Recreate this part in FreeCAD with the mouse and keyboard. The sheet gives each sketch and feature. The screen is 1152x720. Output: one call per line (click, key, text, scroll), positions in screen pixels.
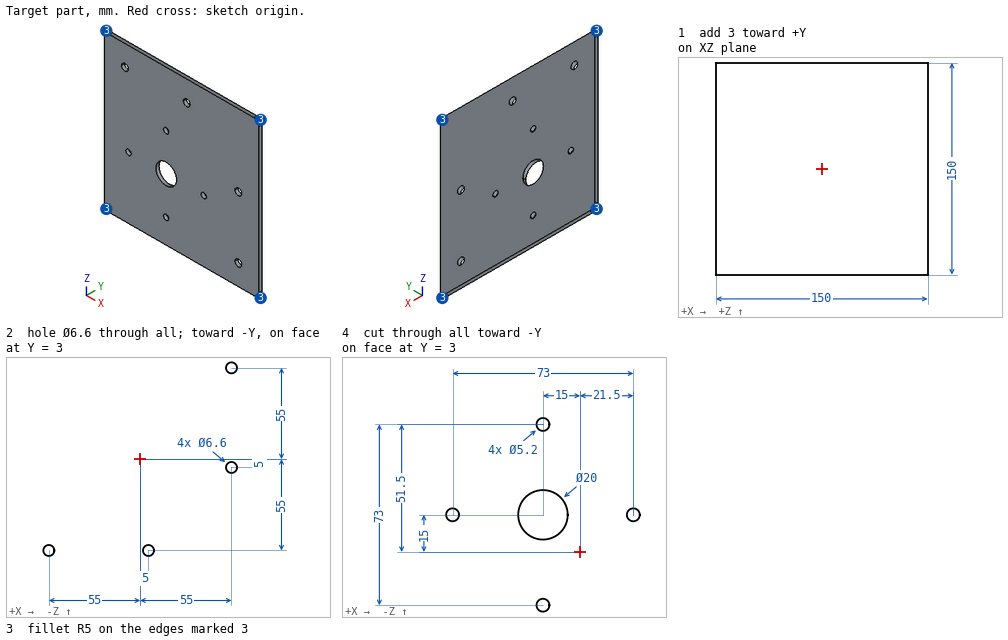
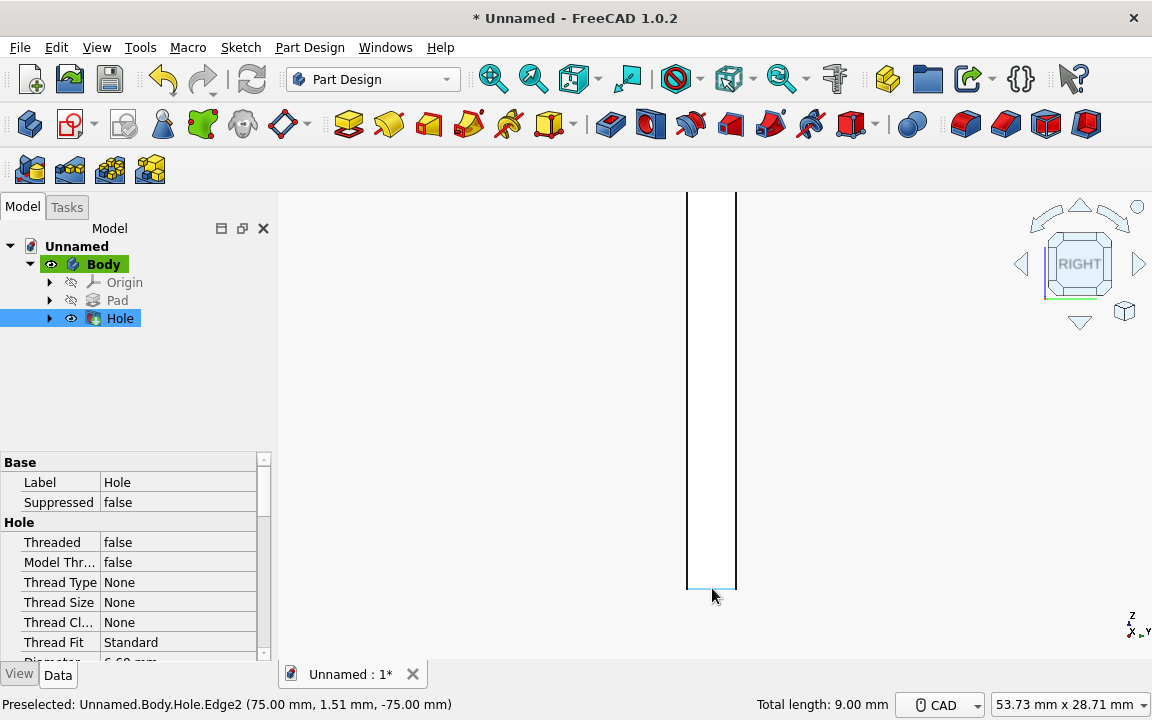
click(494, 80)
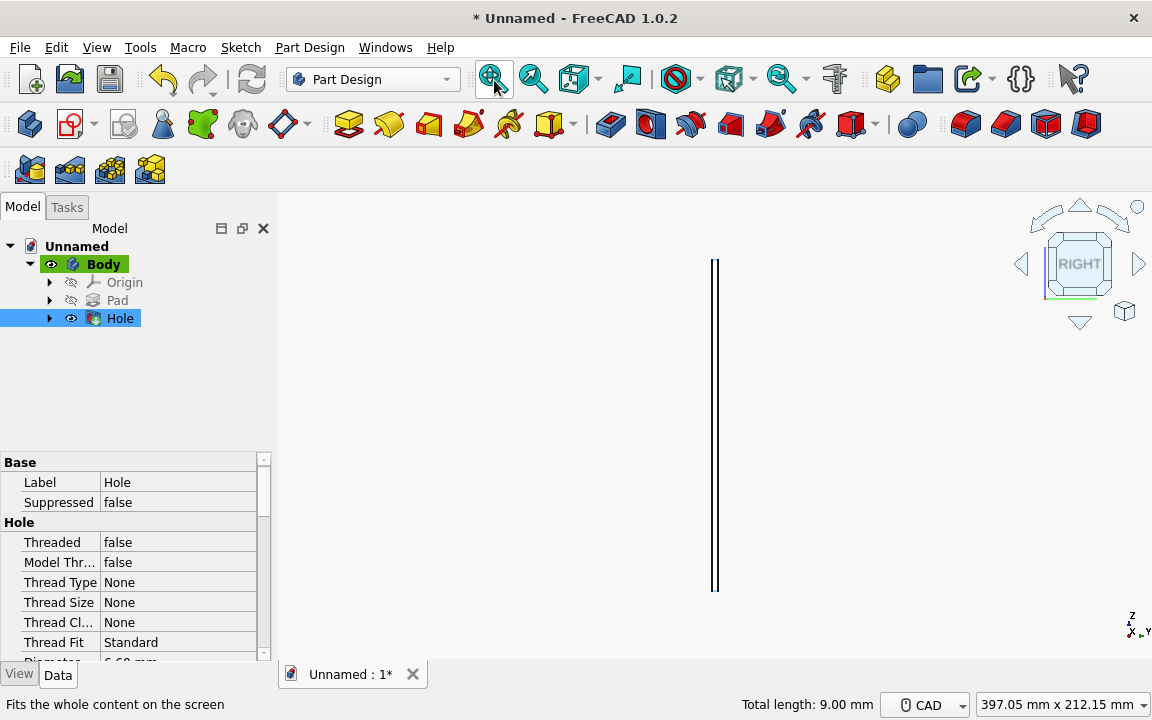
key(5)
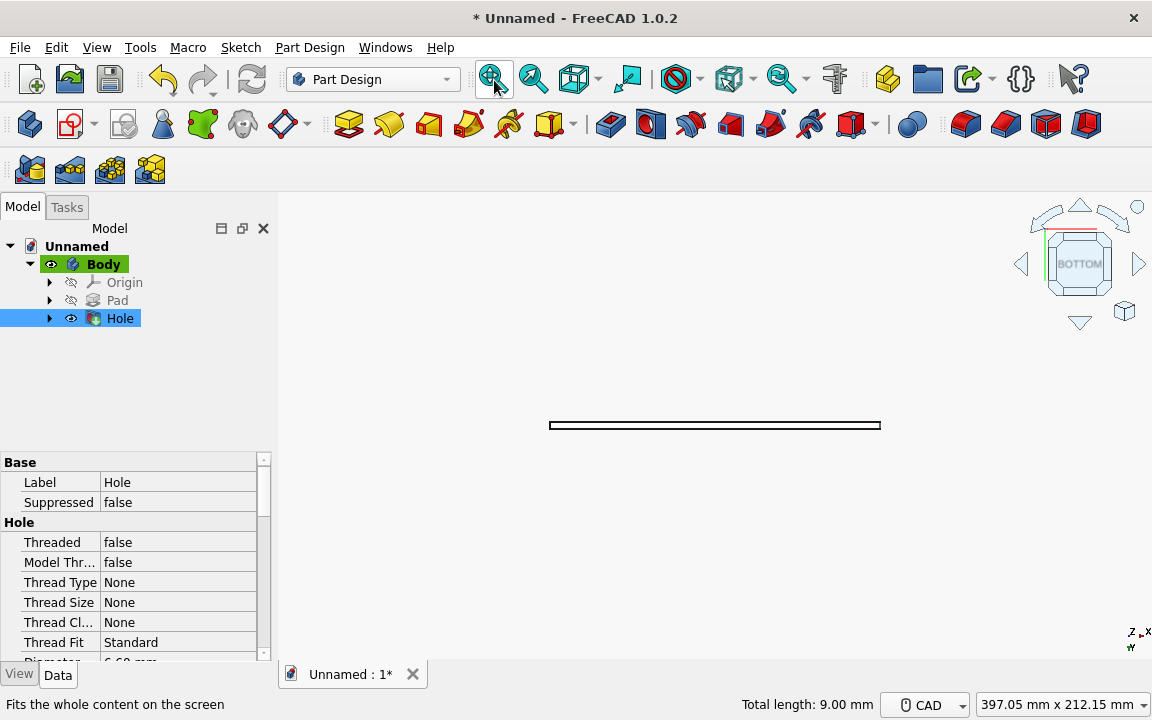
click(494, 80)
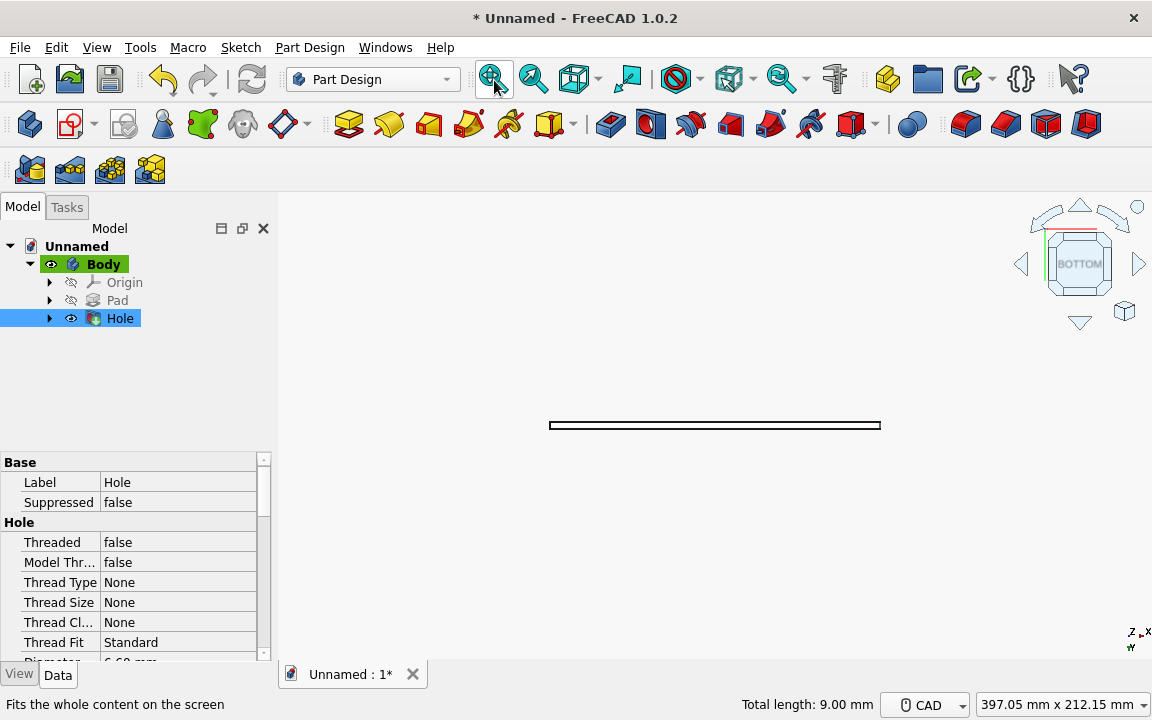
scroll(550, 424, up, 10)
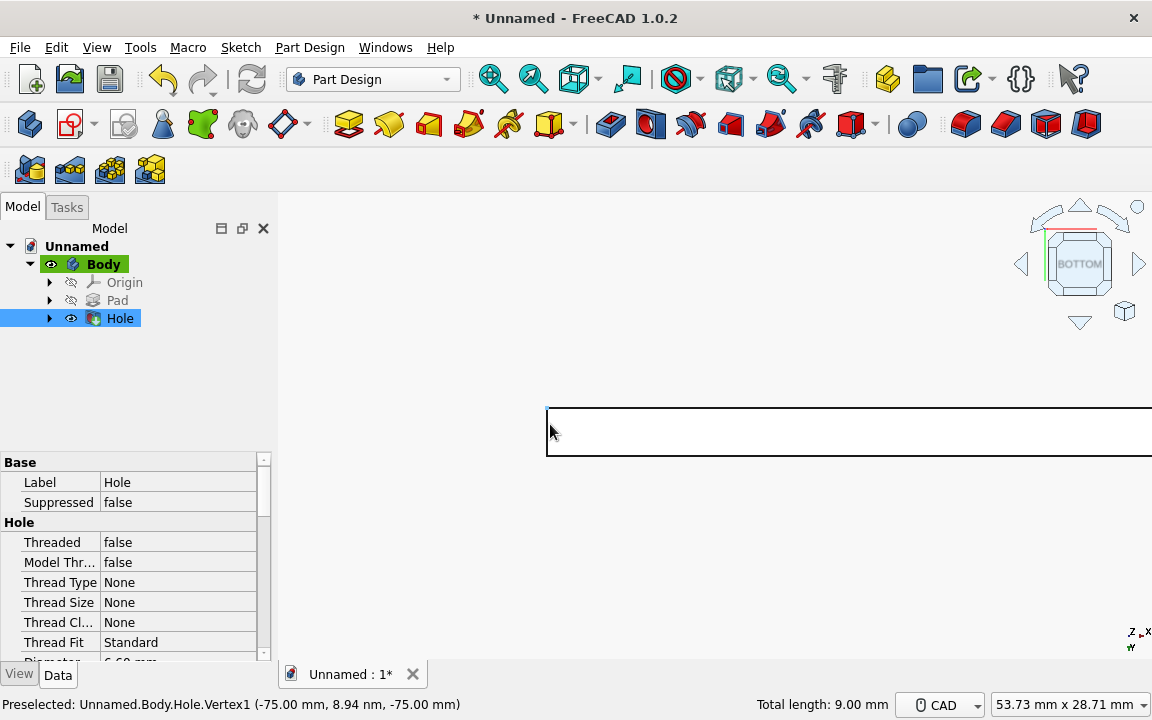
click(547, 431, ctrl)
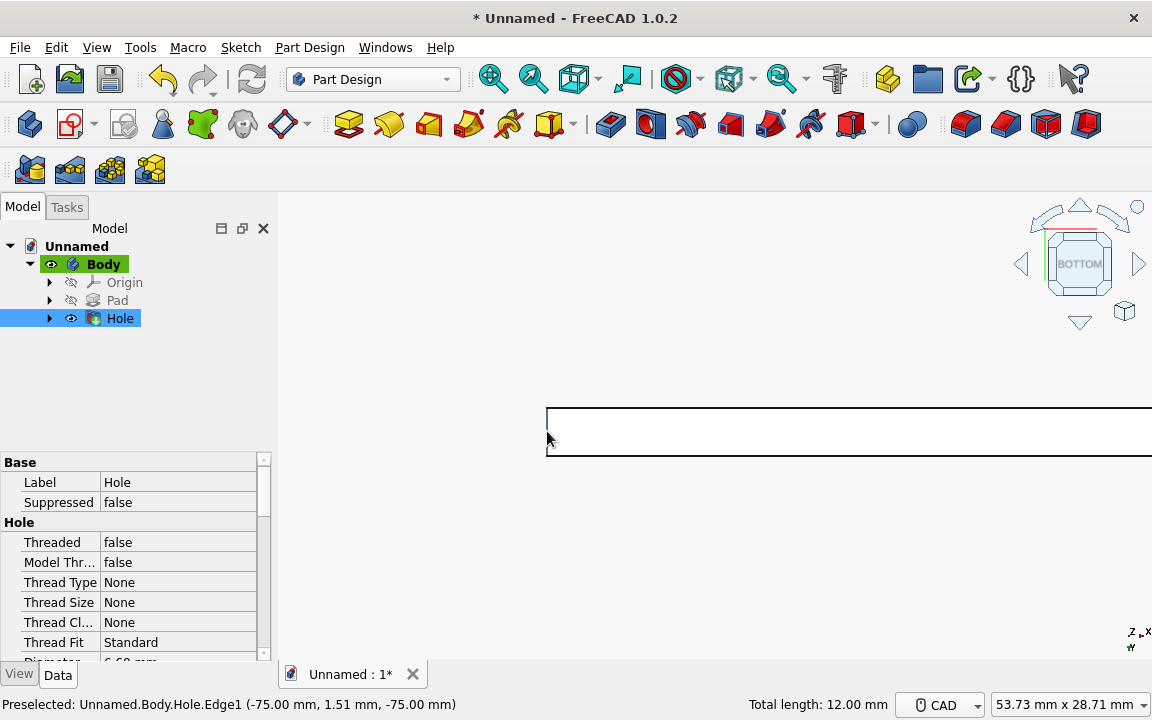
click(966, 124)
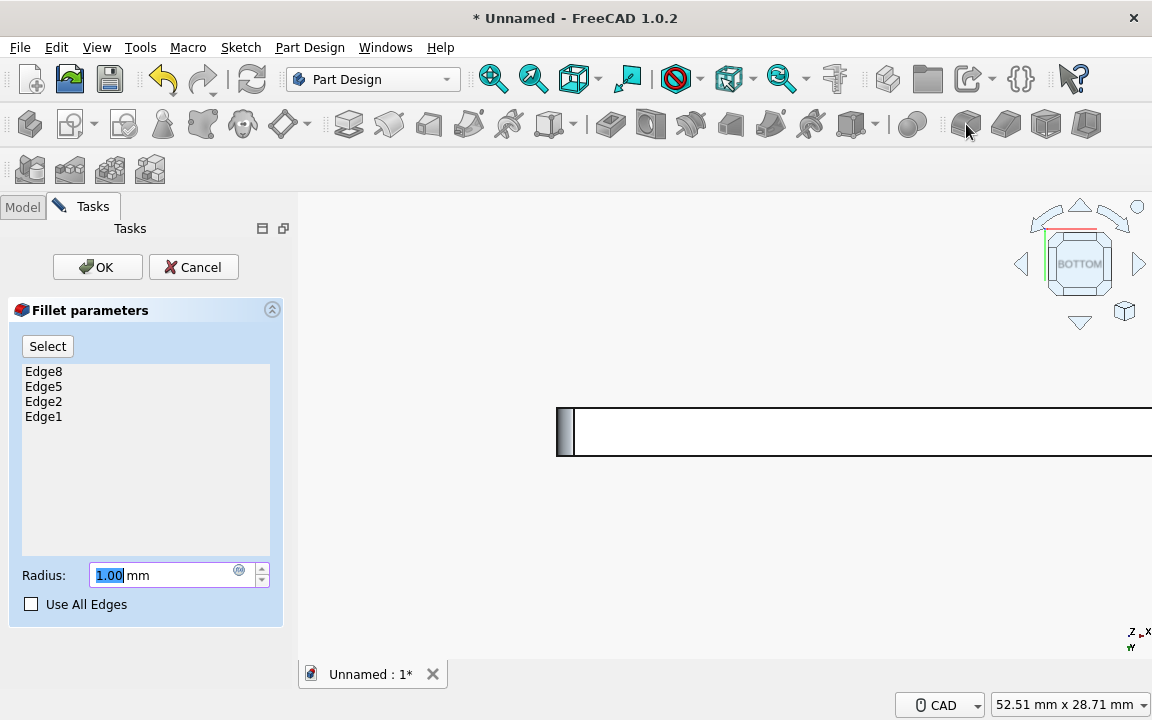
text(5)
key(Tab)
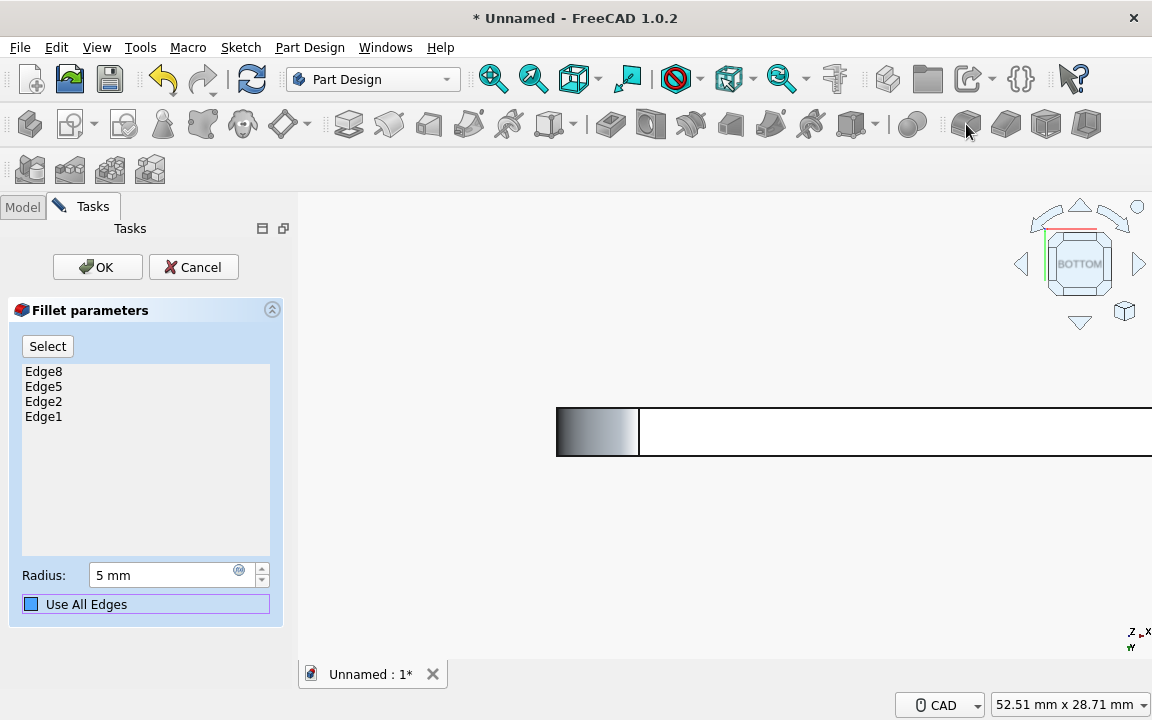
click(98, 267)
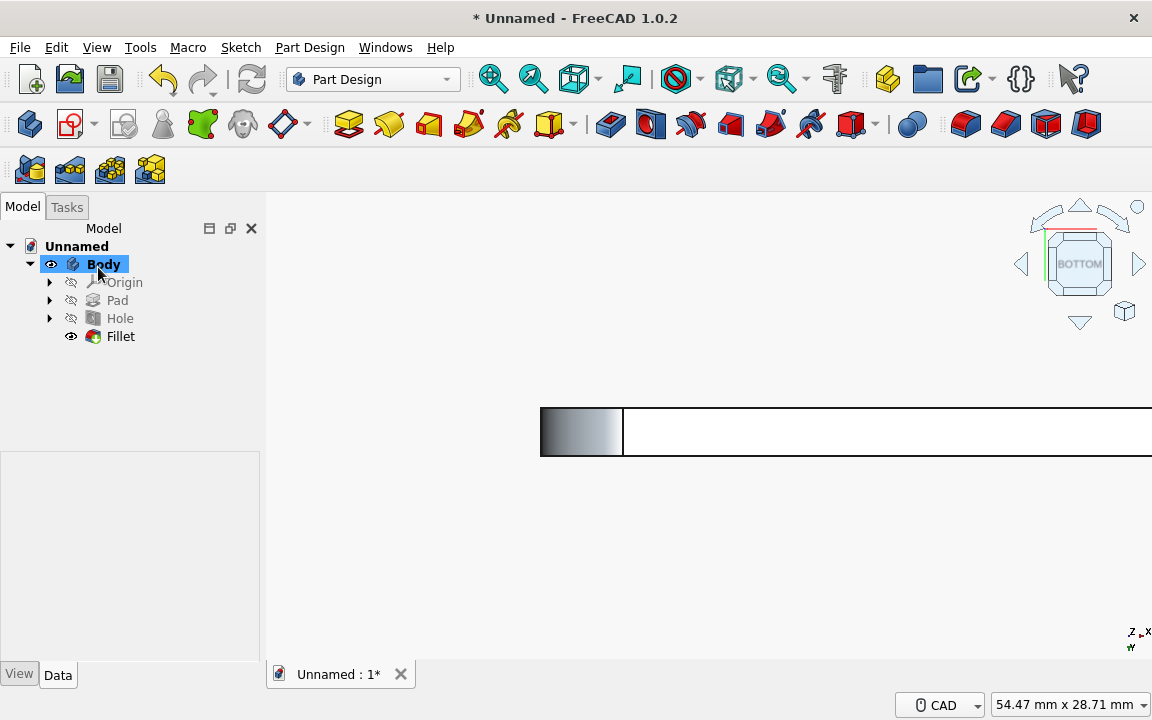
click(494, 80)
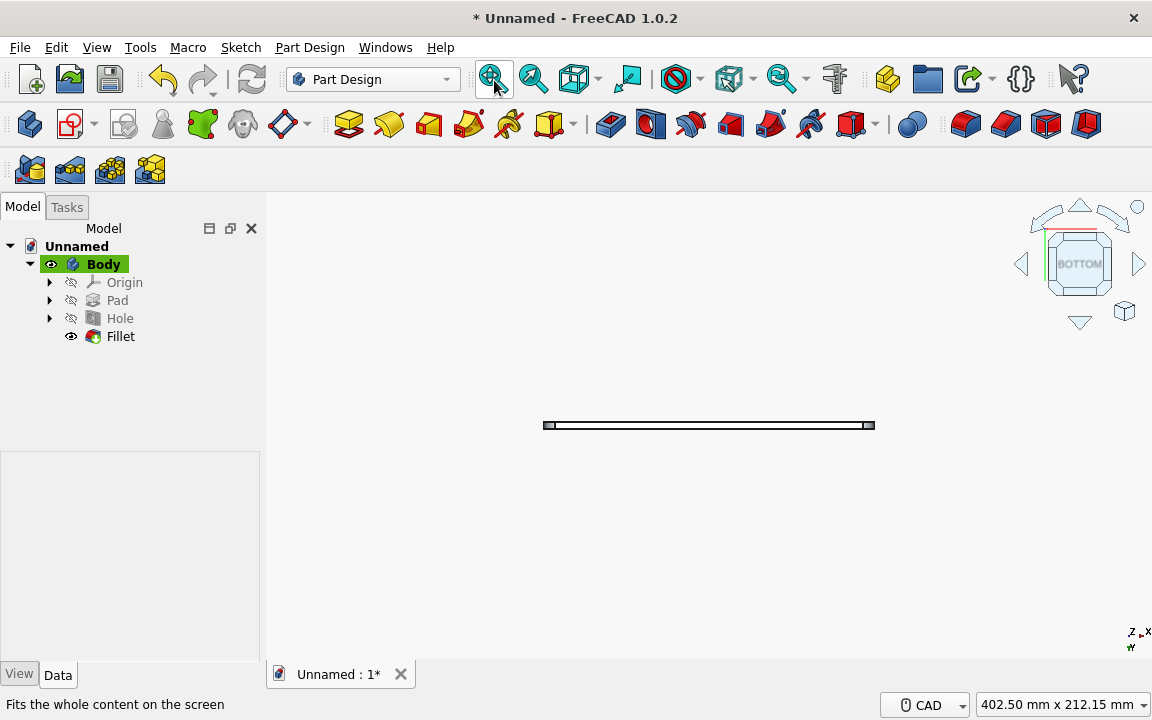
key(4)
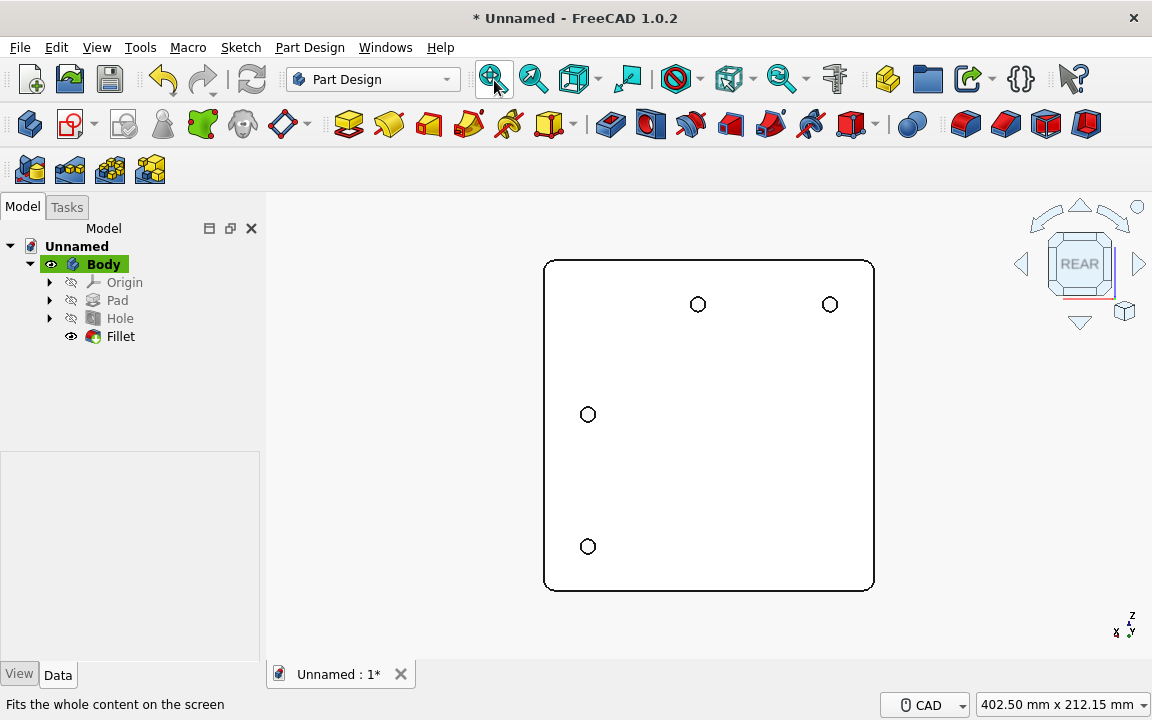
click(709, 472)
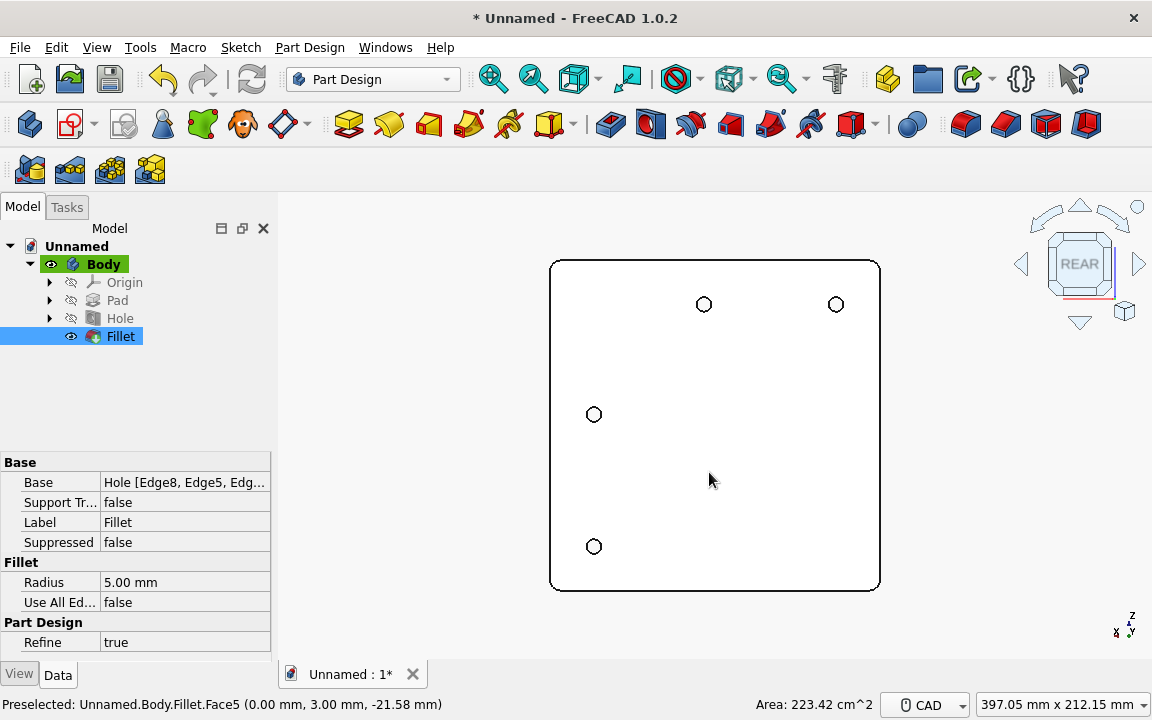
click(70, 124)